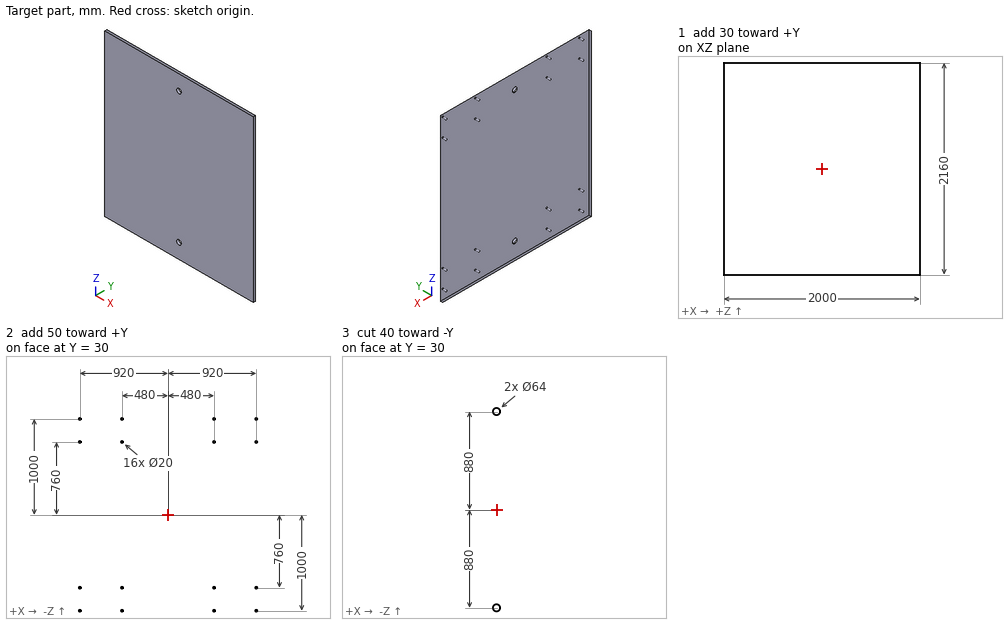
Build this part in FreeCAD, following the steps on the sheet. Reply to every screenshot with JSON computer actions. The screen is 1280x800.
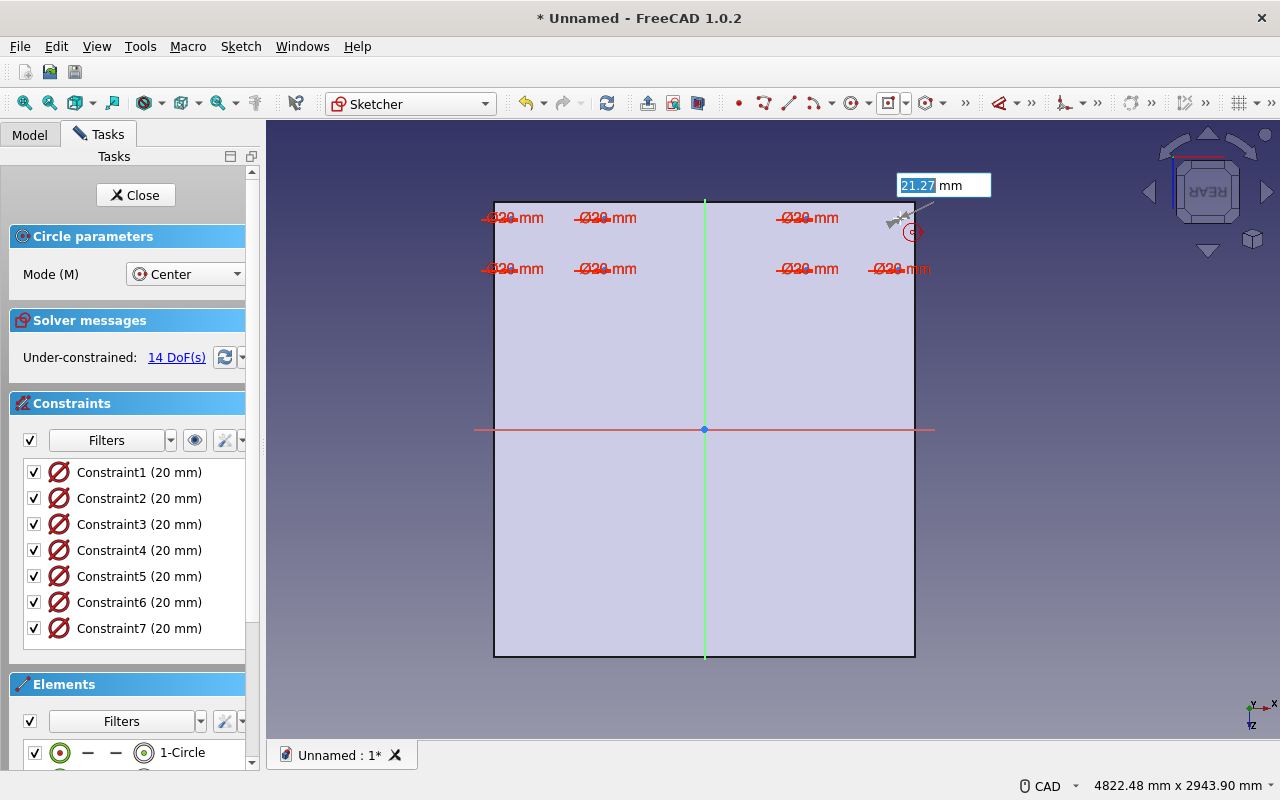
{"action": "type", "text": "20"}
{"action": "key", "text": "Return"}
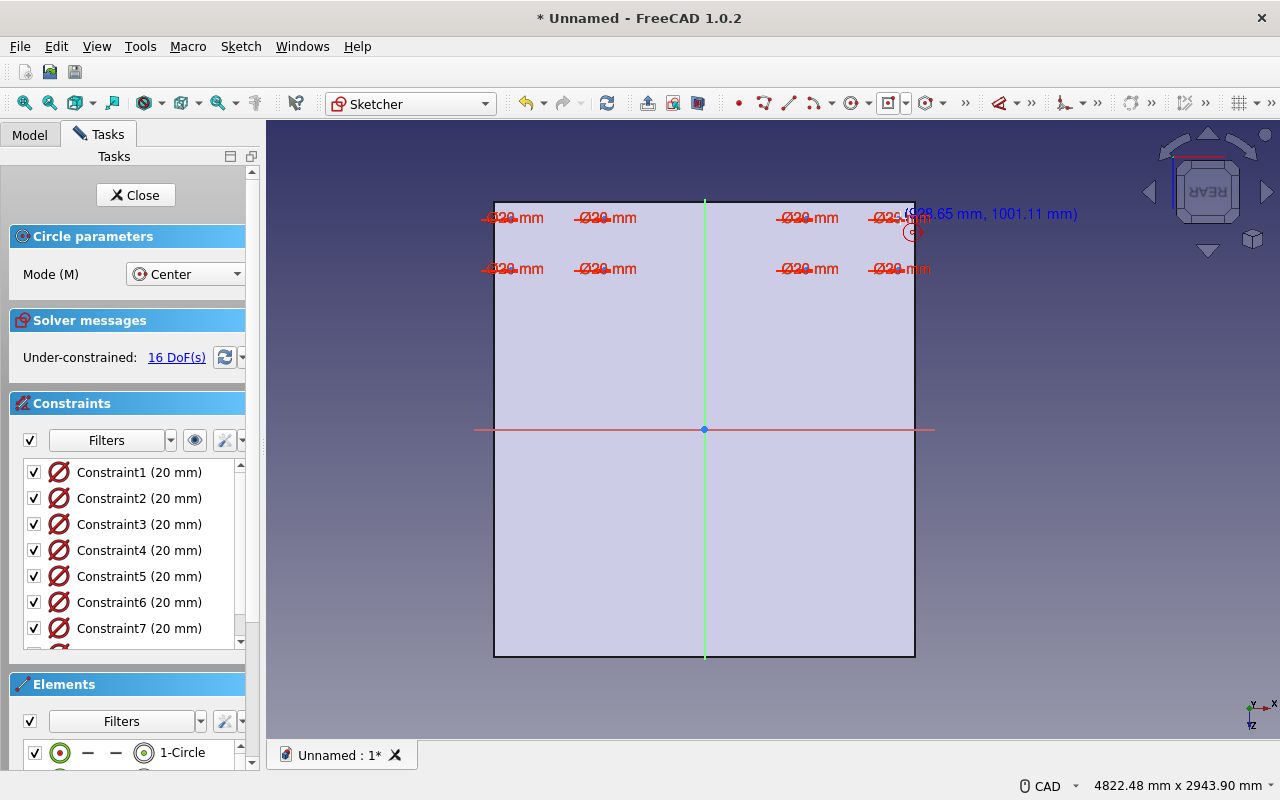
{"action": "scroll", "coordinate": [898, 640], "scroll_direction": "up", "scroll_amount": 12}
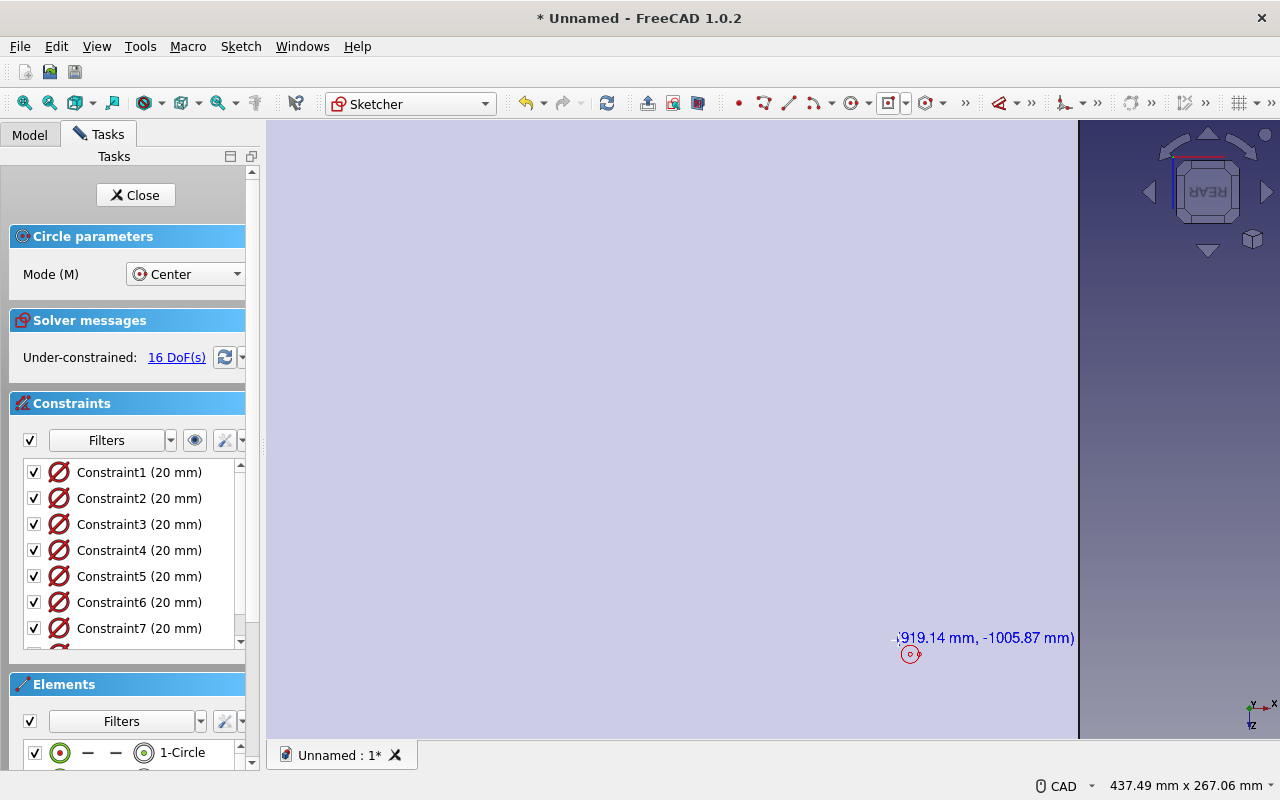
{"action": "scroll", "coordinate": [898, 641], "scroll_direction": "down", "scroll_amount": 12}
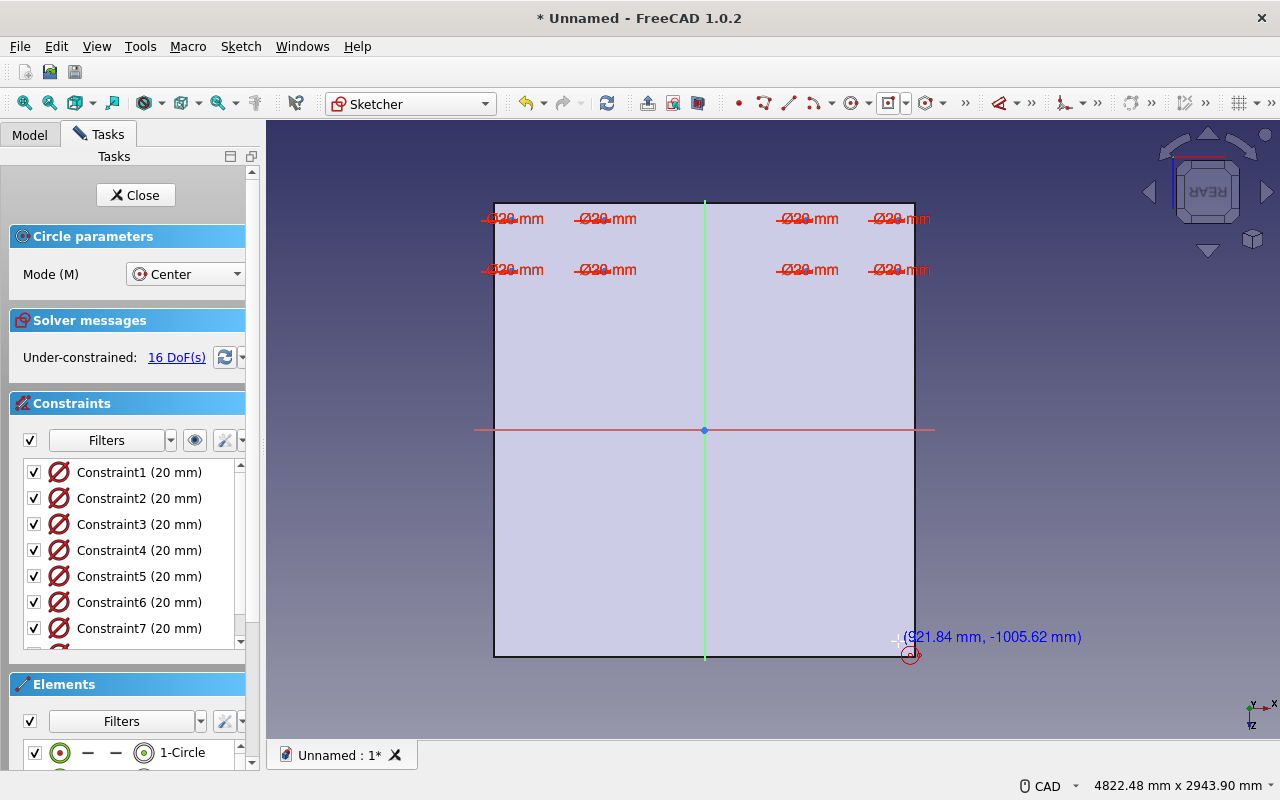
{"action": "left_click", "coordinate": [898, 641]}
{"action": "mouse_move", "coordinate": [900, 639]}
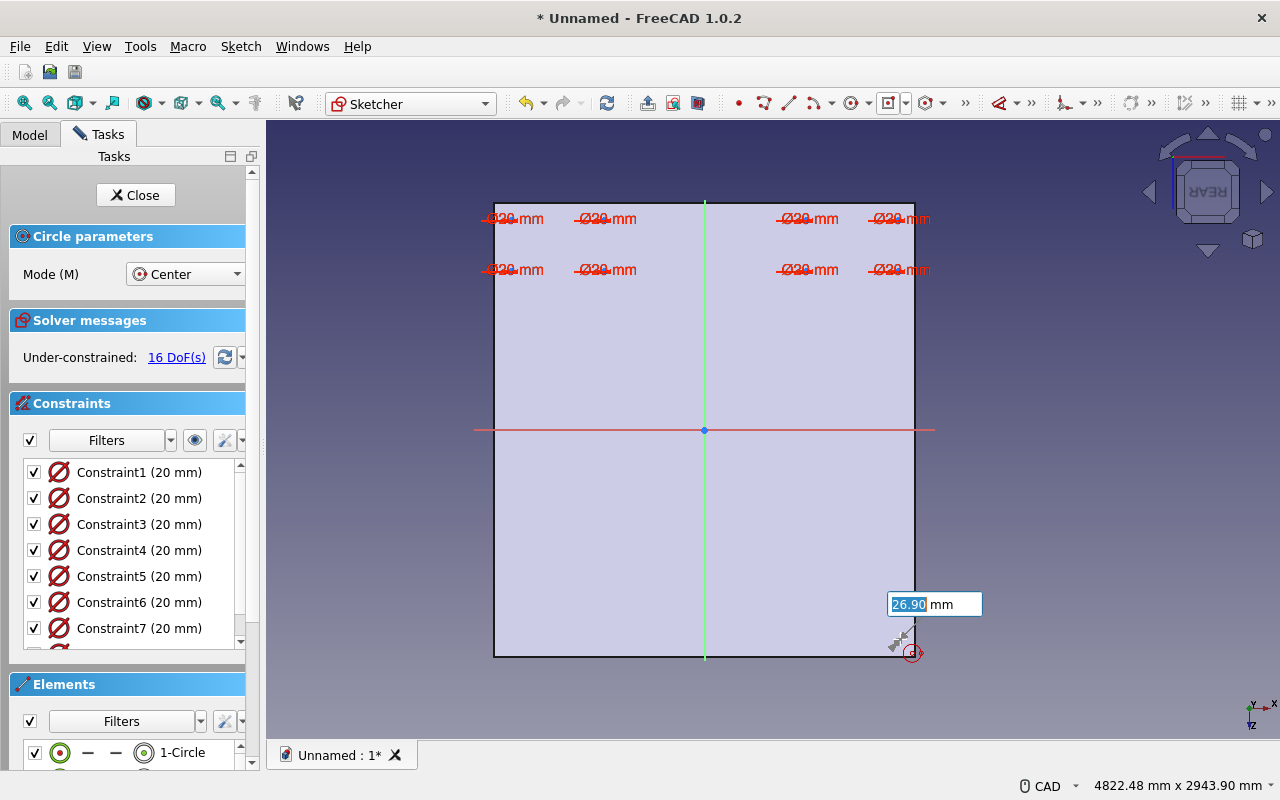
{"action": "type", "text": "20"}
{"action": "key", "text": "Return"}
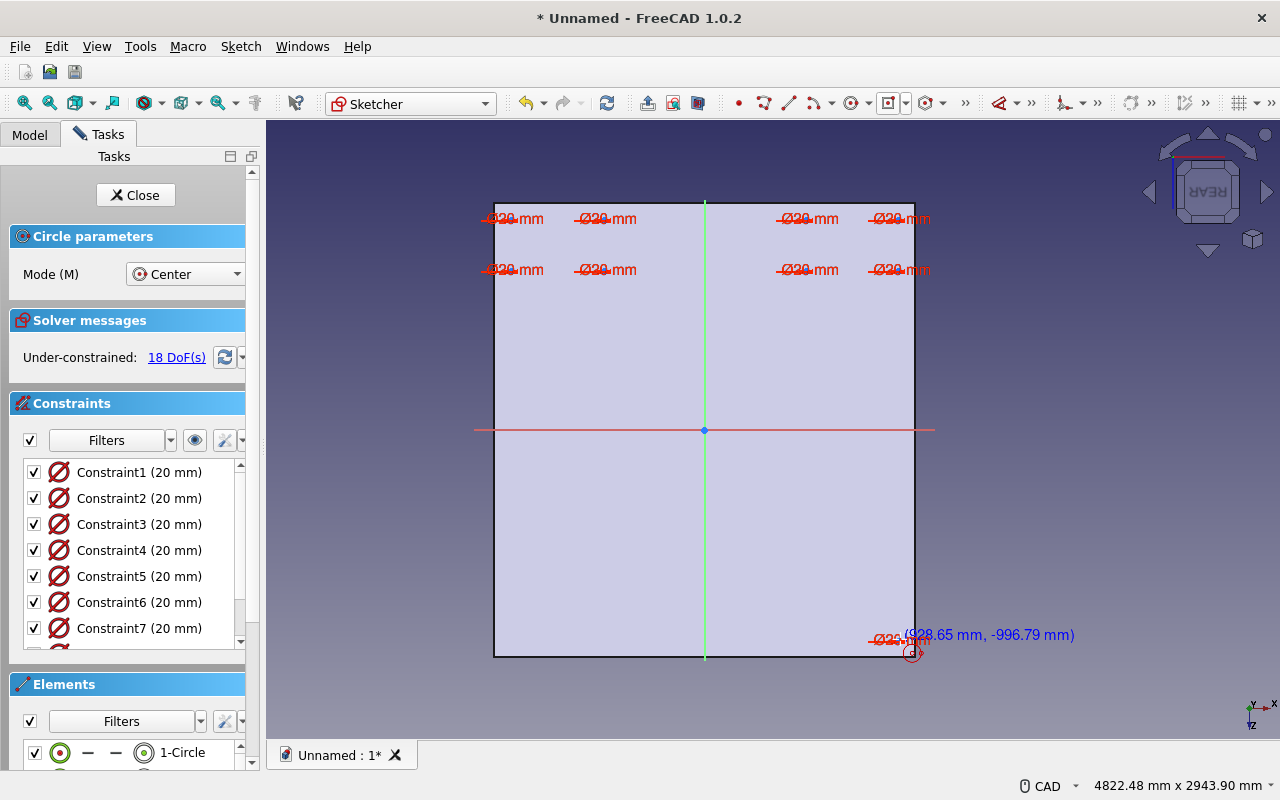
{"action": "scroll", "coordinate": [898, 590], "scroll_direction": "up", "scroll_amount": 12}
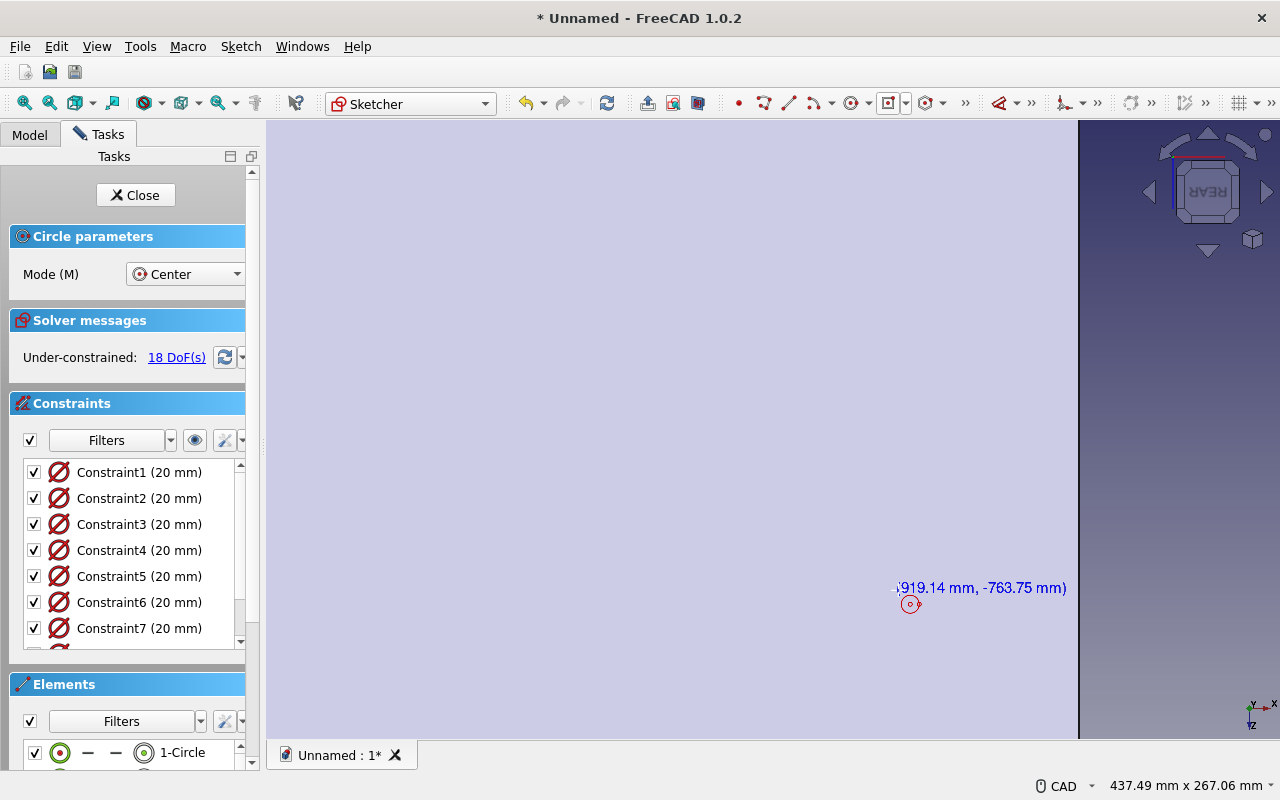
{"action": "scroll", "coordinate": [898, 590], "scroll_direction": "down", "scroll_amount": 12}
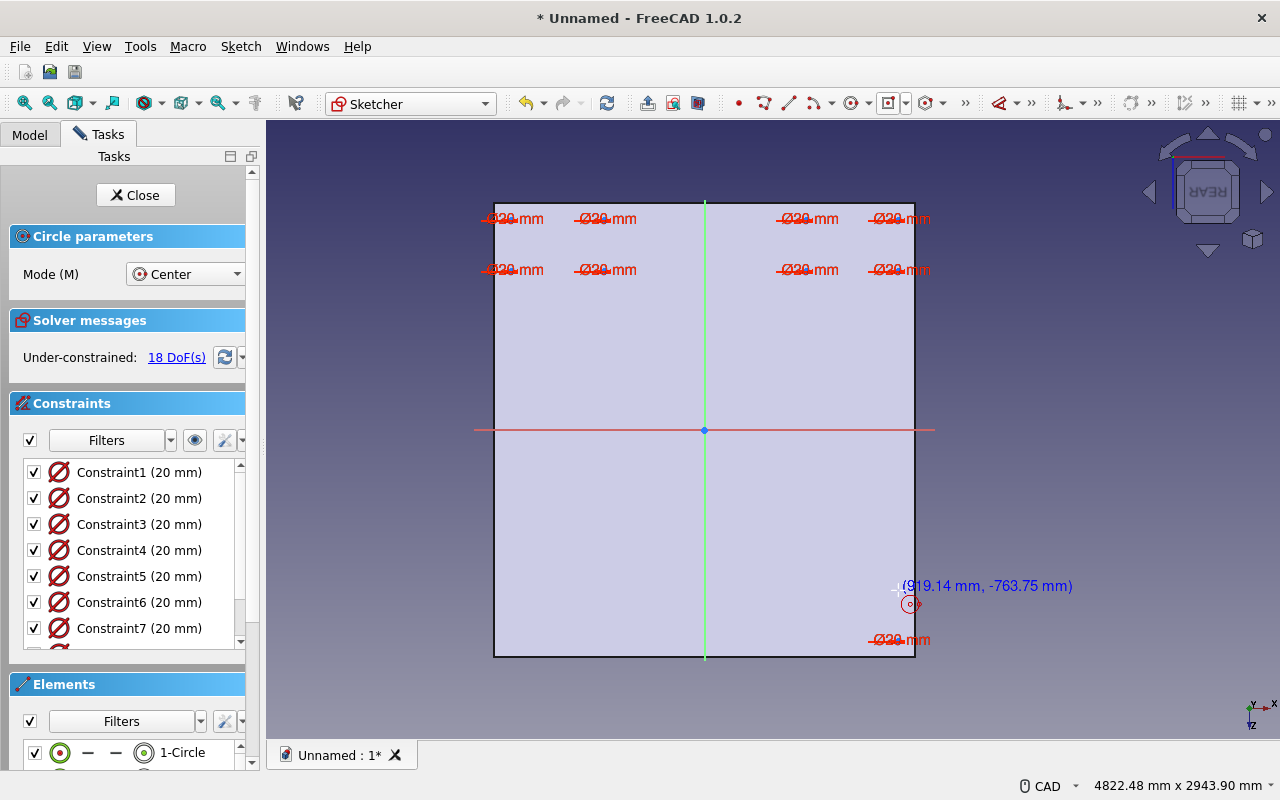
{"action": "left_click", "coordinate": [898, 590]}
{"action": "mouse_move", "coordinate": [900, 589]}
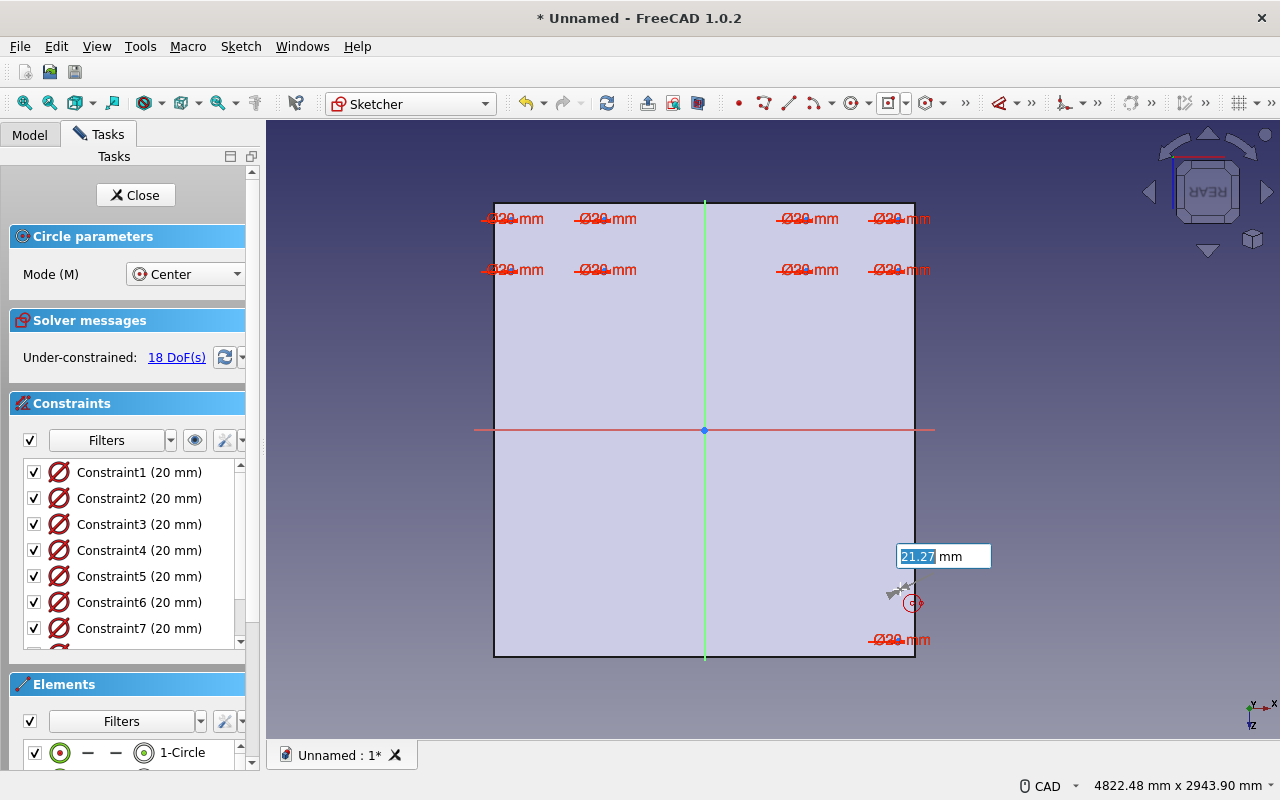
{"action": "type", "text": "20"}
{"action": "key", "text": "Return"}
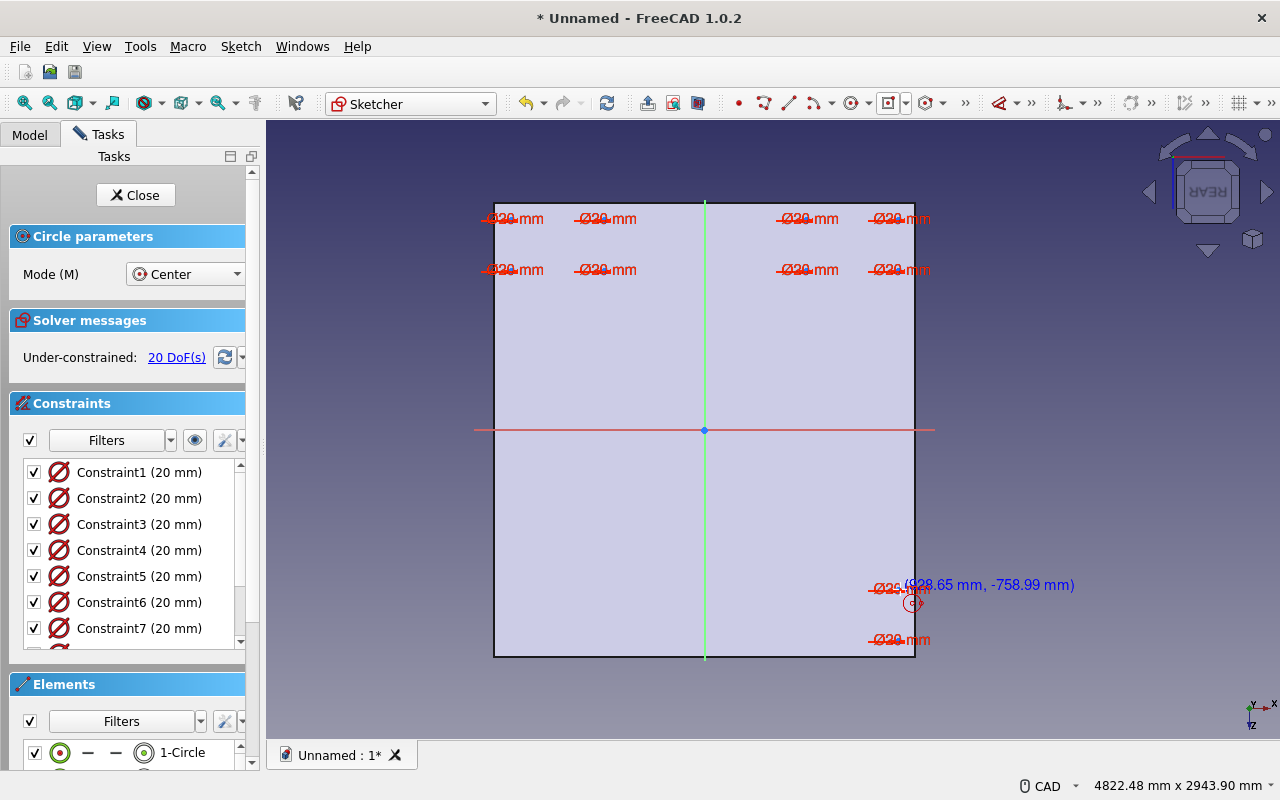
{"action": "scroll", "coordinate": [806, 641], "scroll_direction": "up", "scroll_amount": 12}